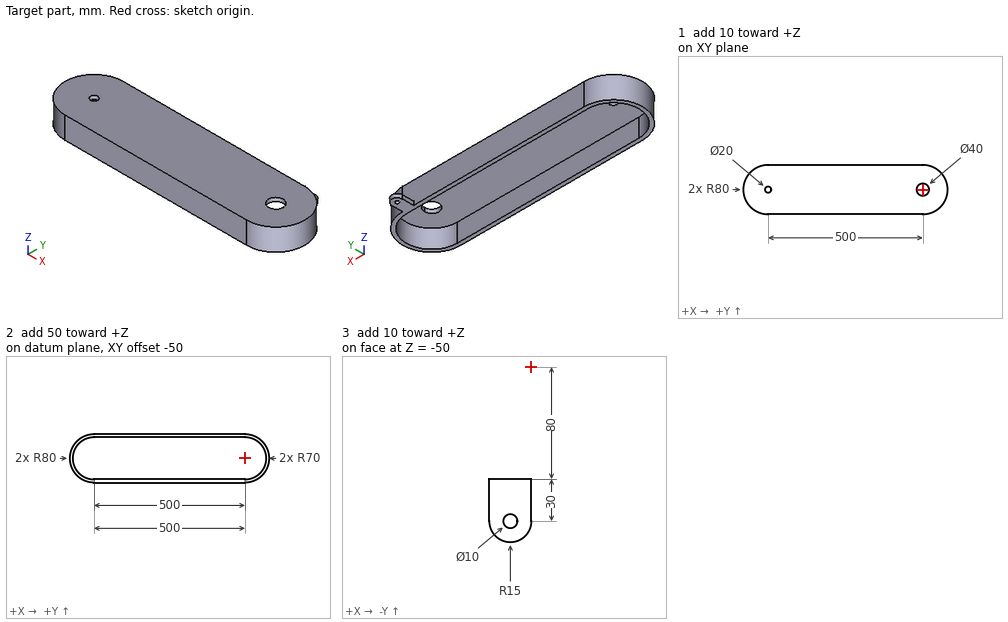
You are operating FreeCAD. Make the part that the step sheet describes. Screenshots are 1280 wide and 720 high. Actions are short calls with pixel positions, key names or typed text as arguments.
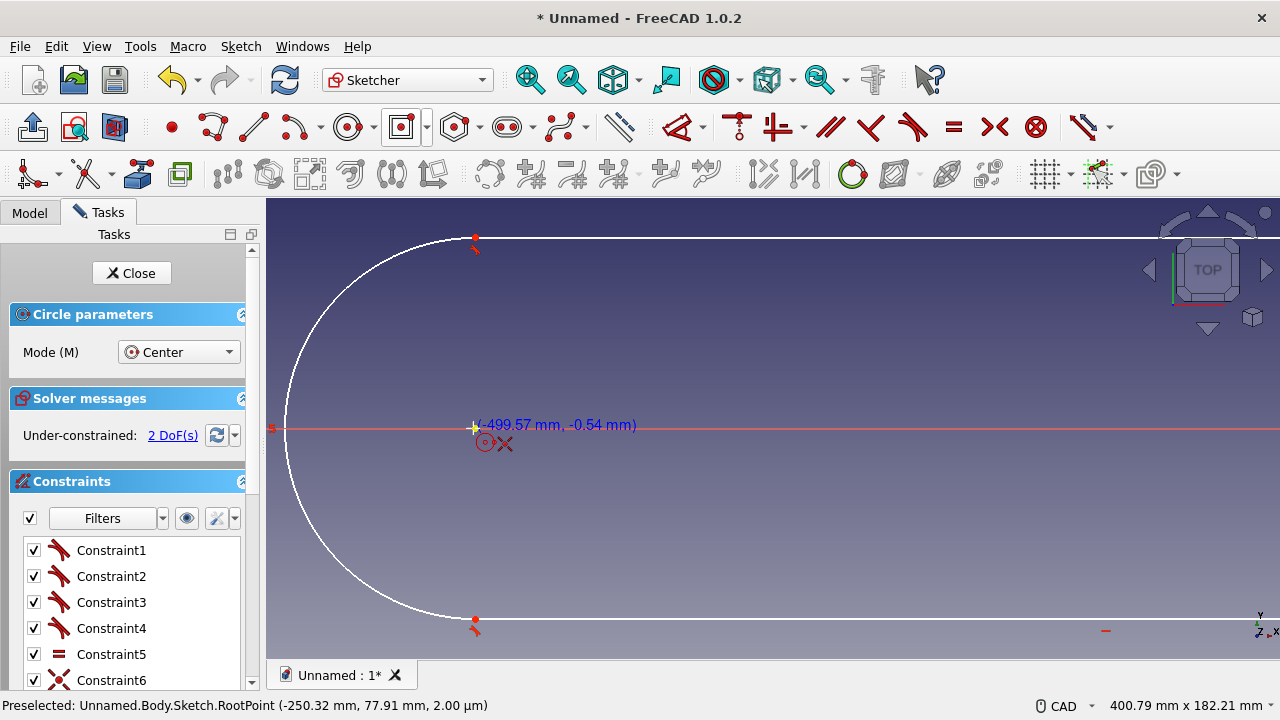
click(473, 405)
move(489, 411)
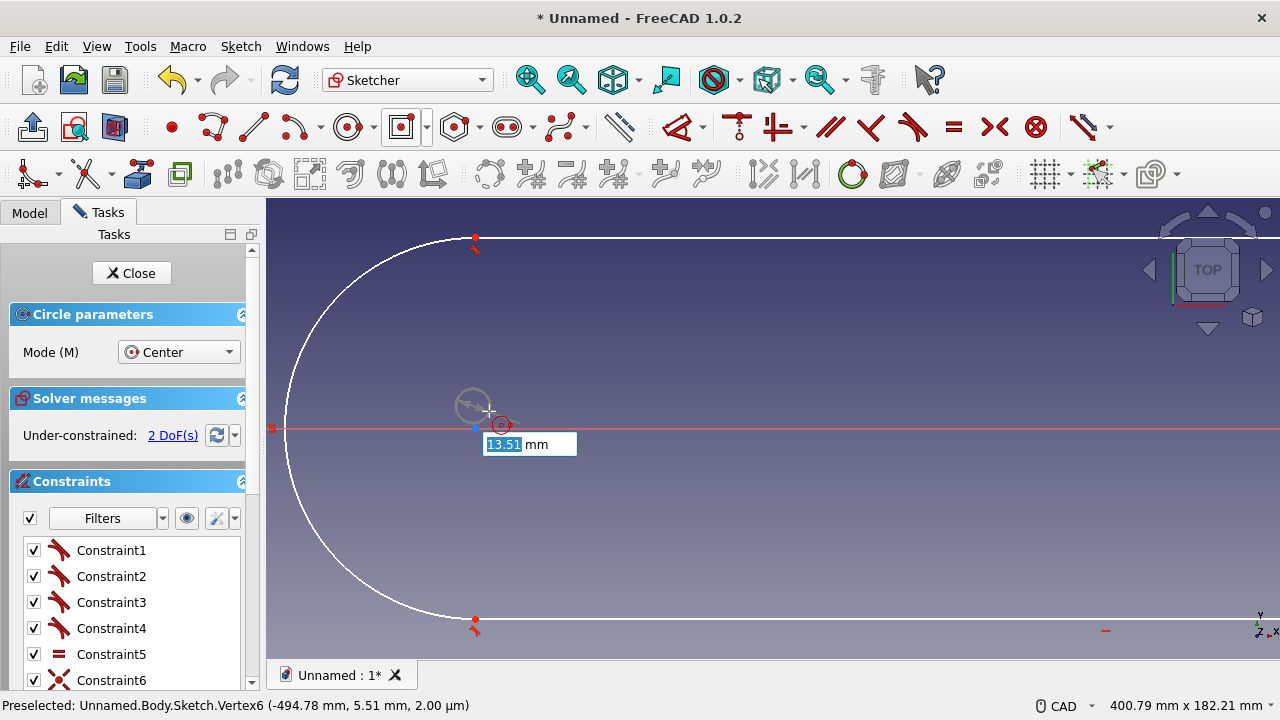
text(20)
key(Return)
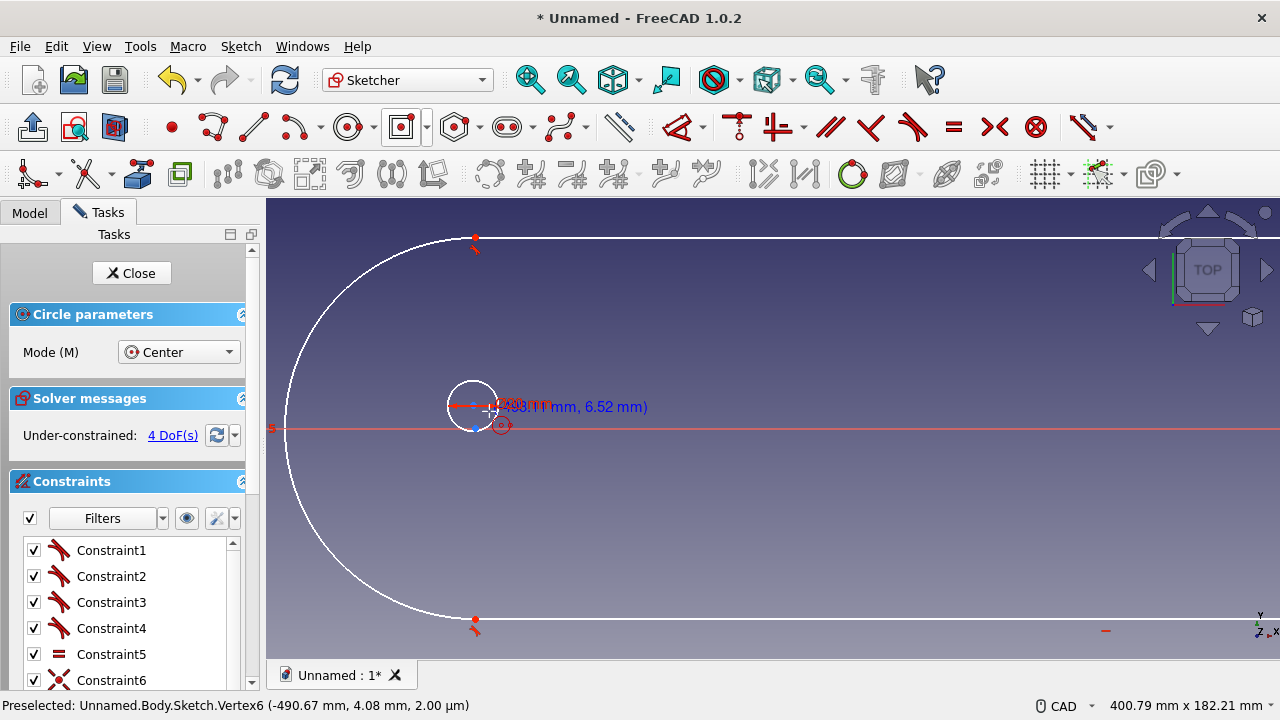
scroll(472, 428, down, 5)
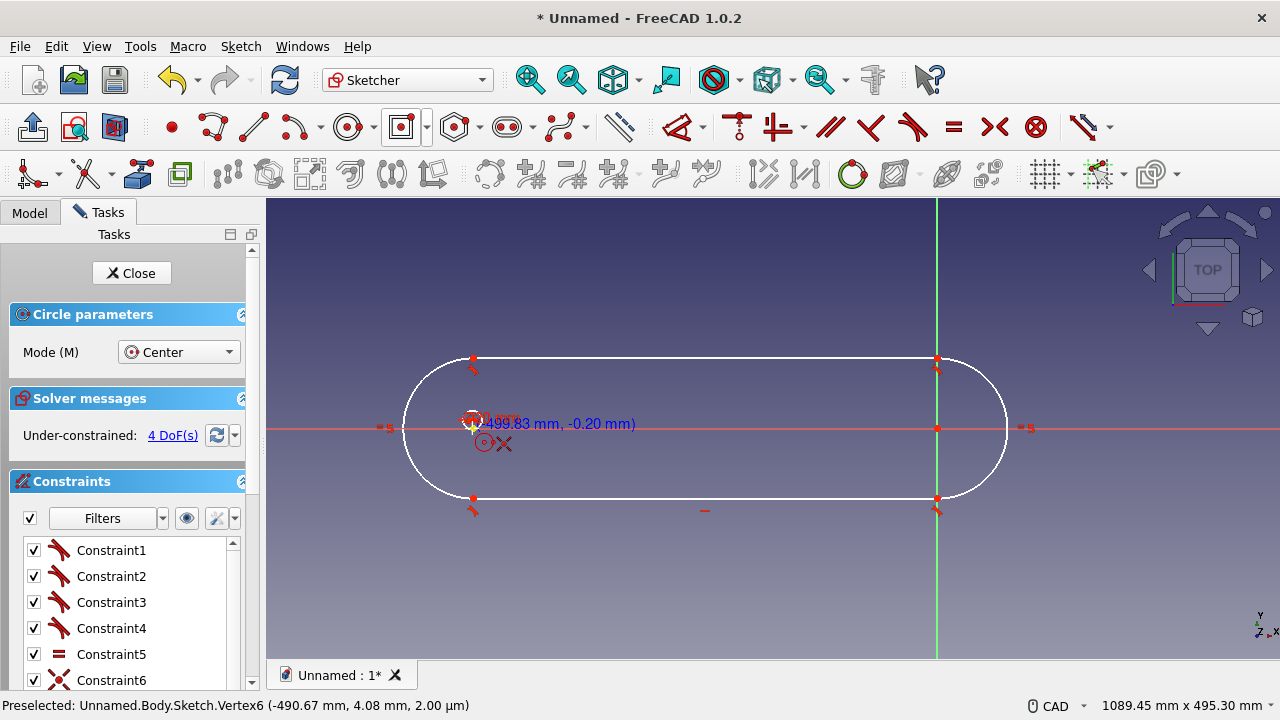
click(937, 428)
move(951, 415)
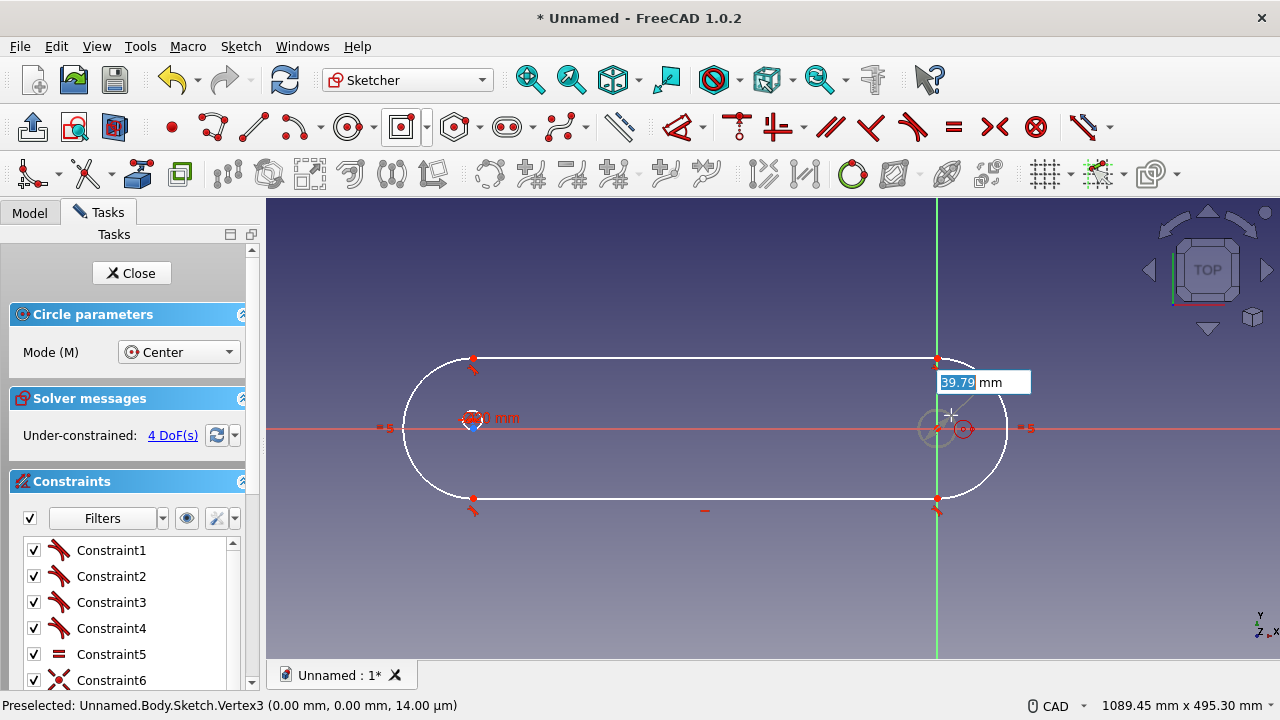
text(40)
key(Return)
key(Escape)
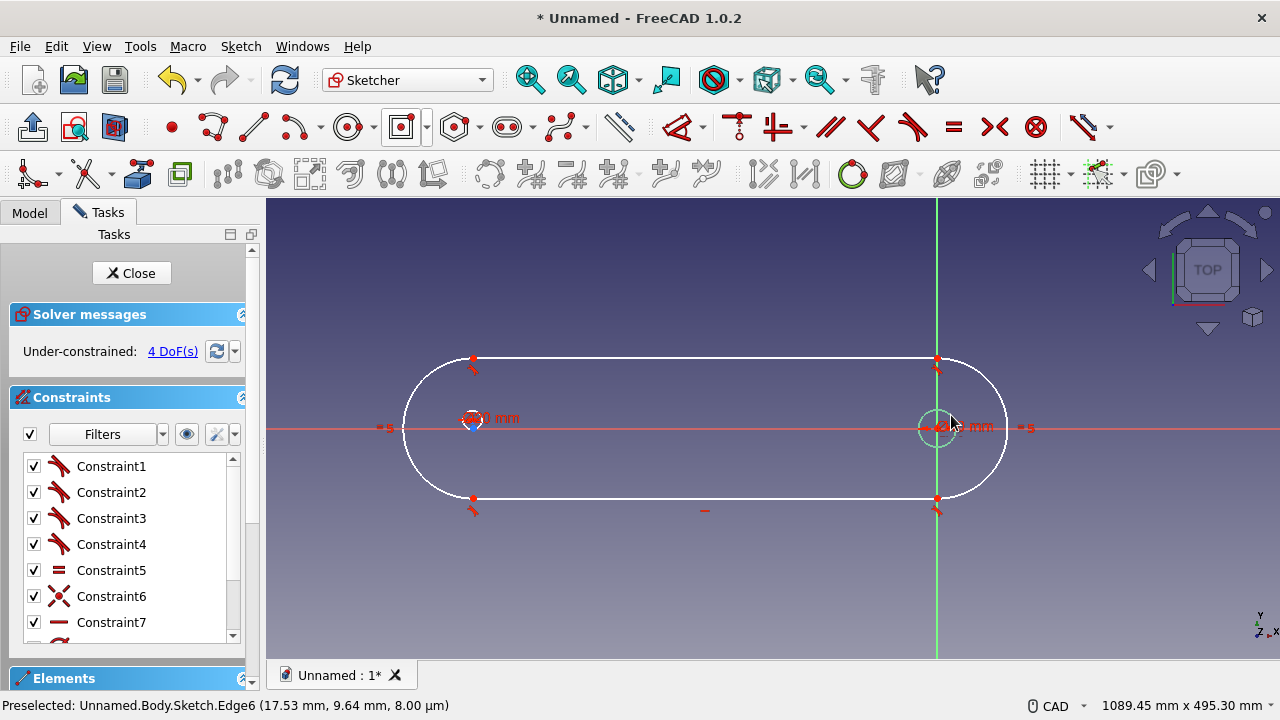
scroll(479, 414, up, 2)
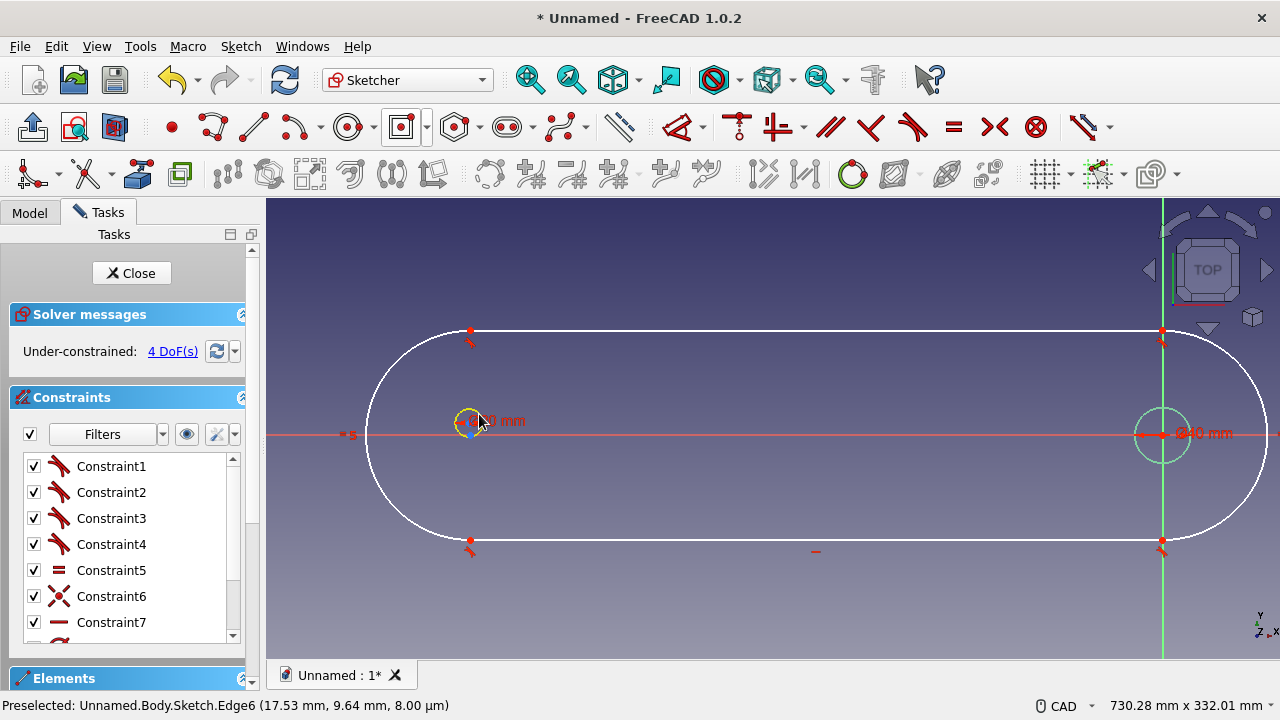
click(479, 413)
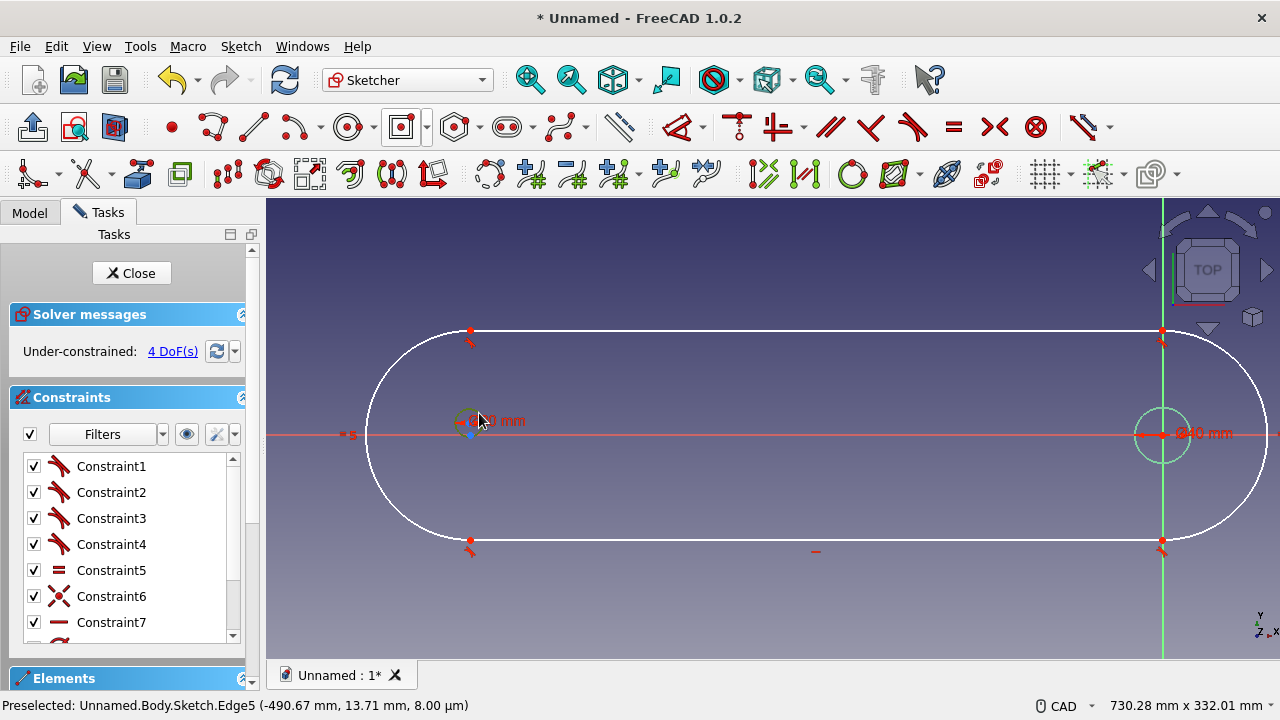
click(386, 374)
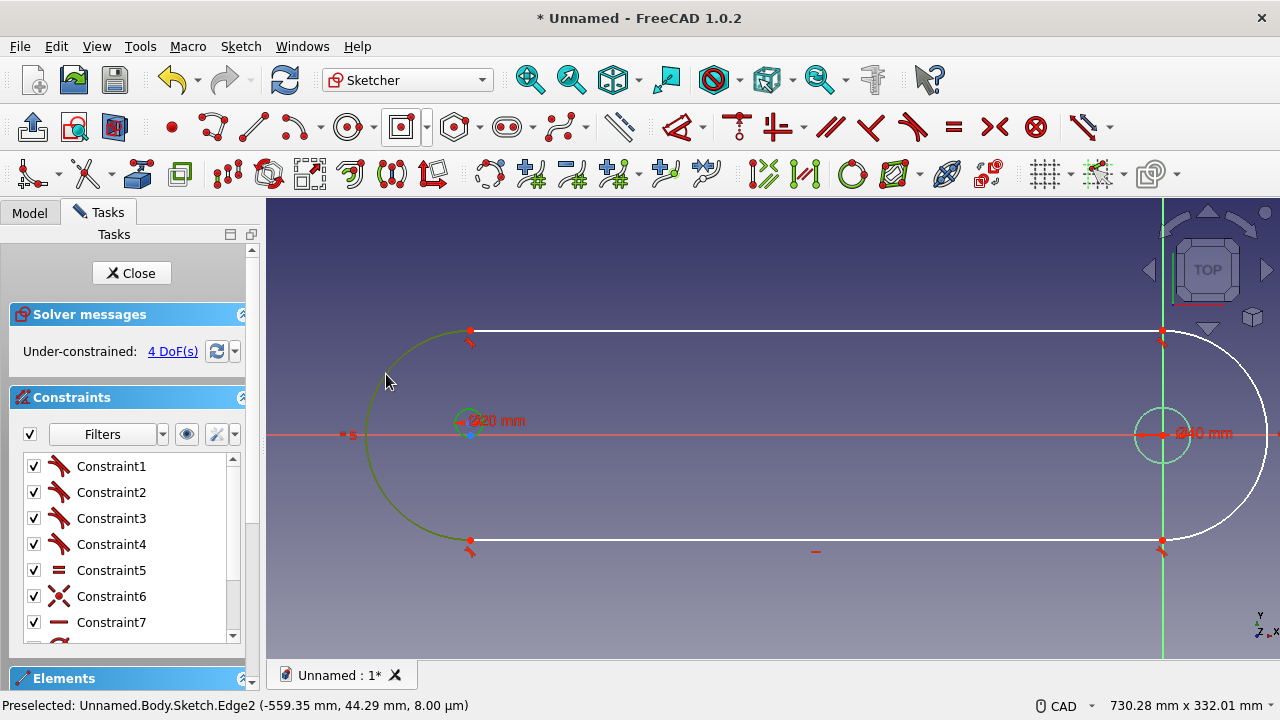
click(737, 128)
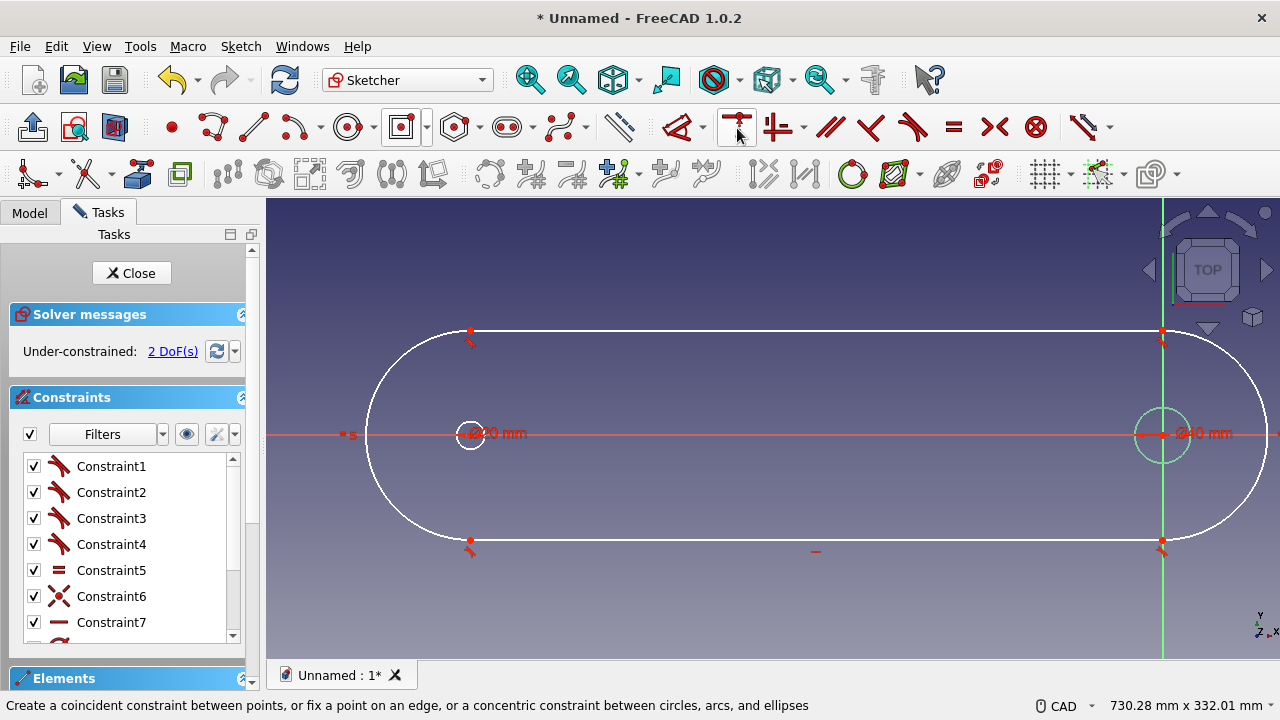
click(676, 128)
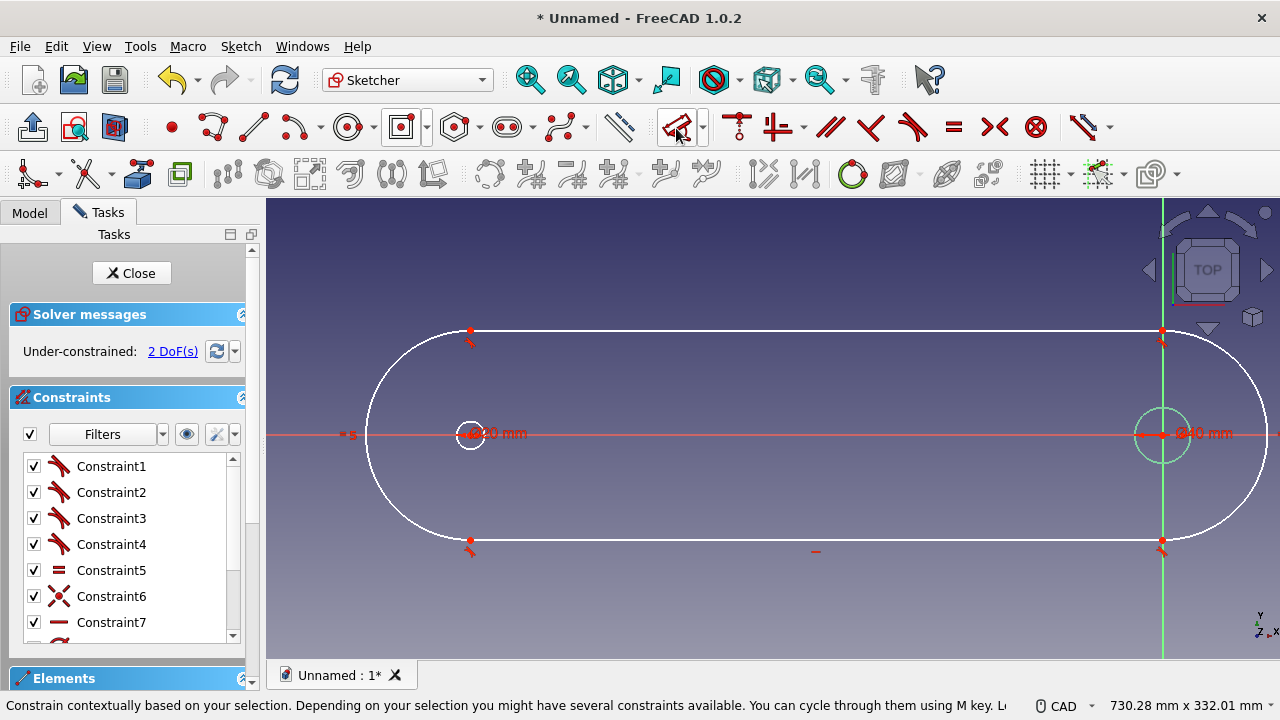
scroll(479, 414, down, 2)